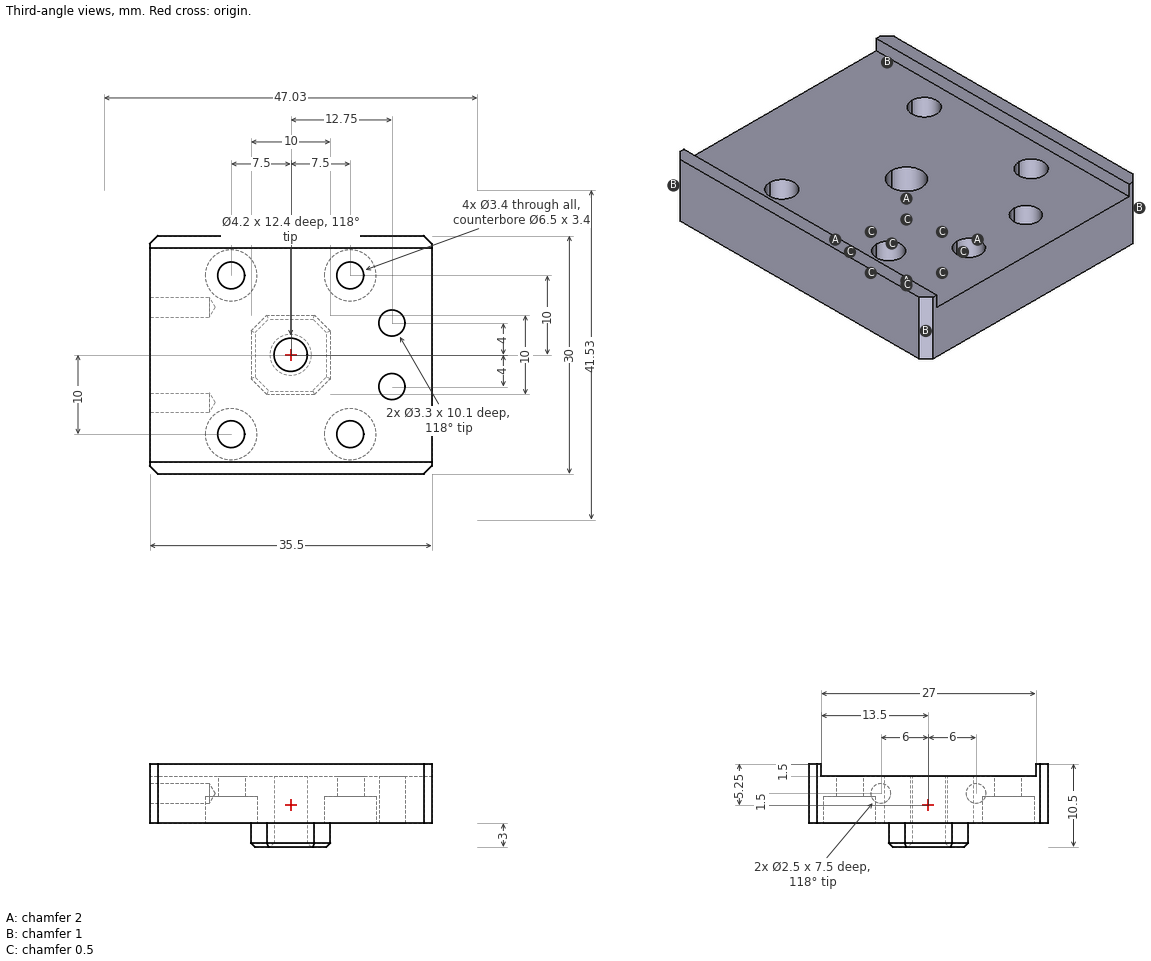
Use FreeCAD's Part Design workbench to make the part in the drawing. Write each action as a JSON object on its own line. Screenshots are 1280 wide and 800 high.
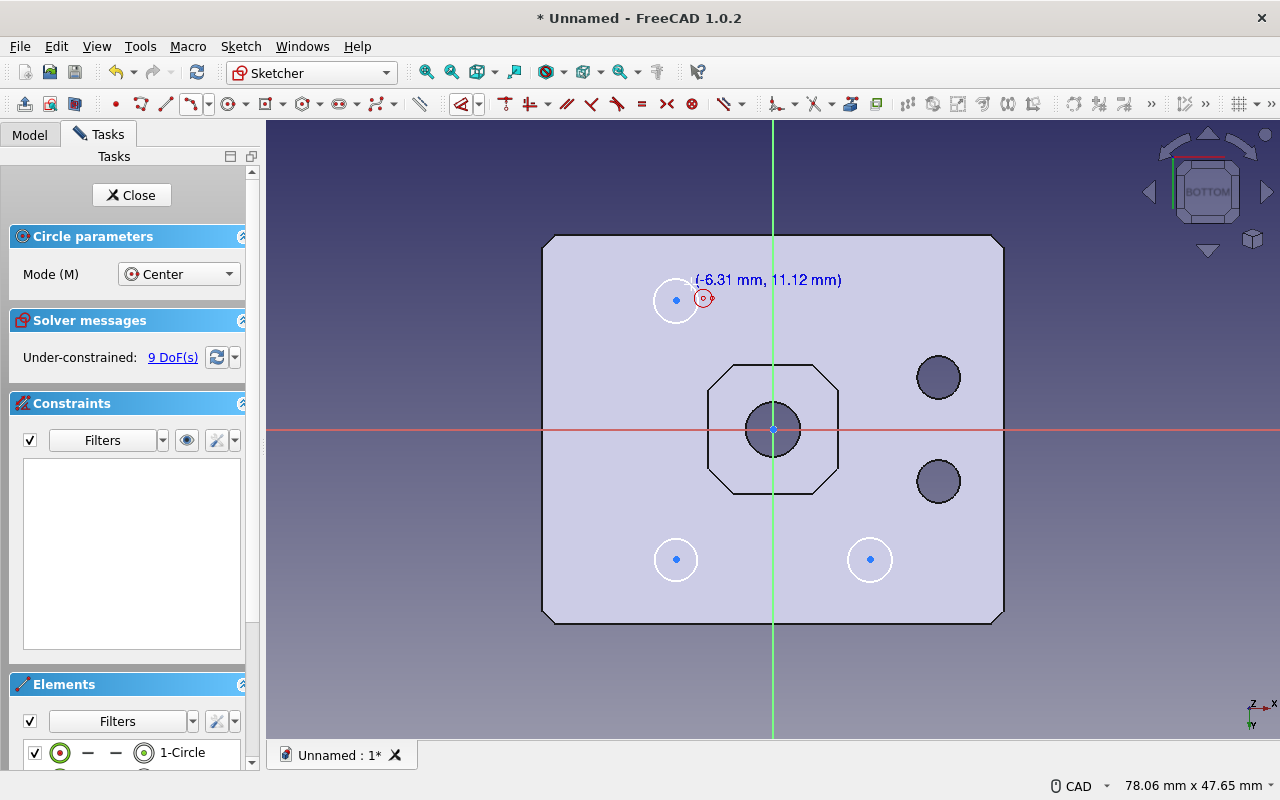
{"action": "left_click", "coordinate": [870, 300]}
{"action": "left_click", "coordinate": [886, 284]}
{"action": "key", "text": "Escape"}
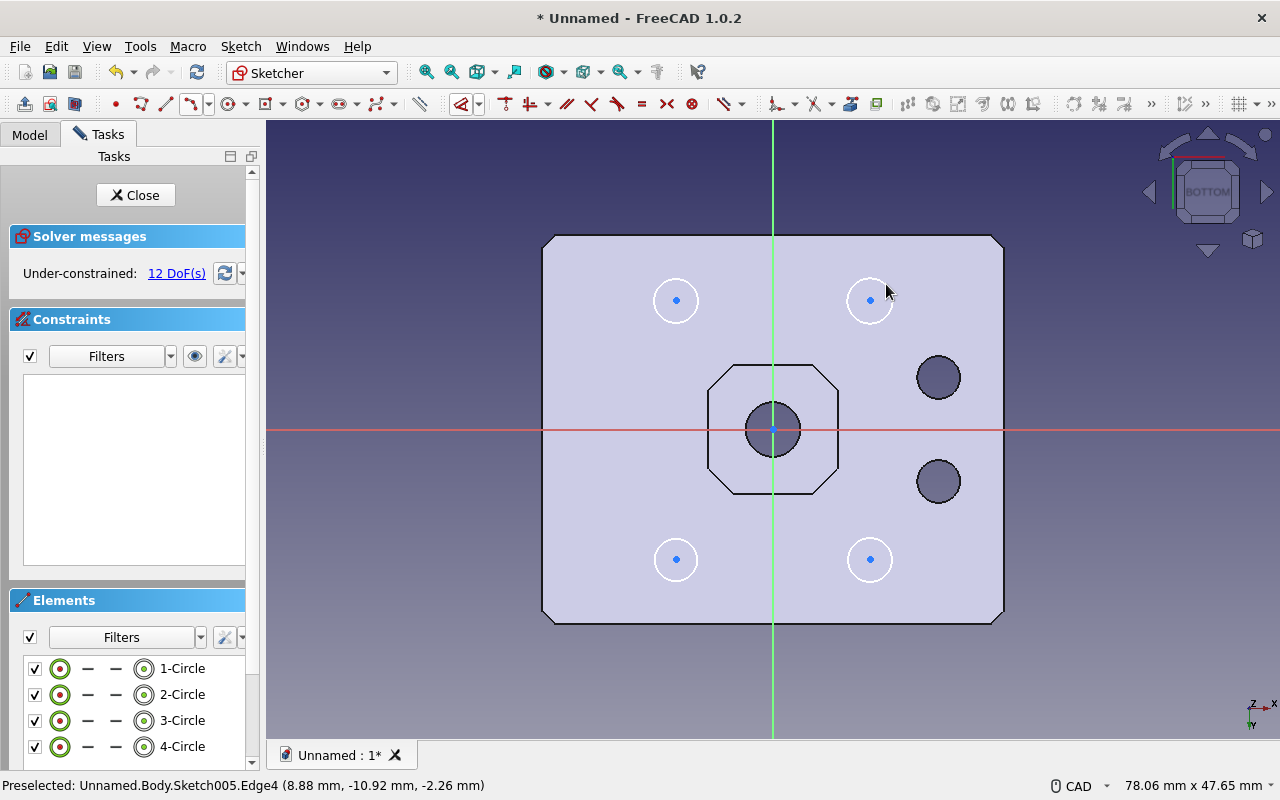
{"action": "left_click", "coordinate": [885, 544]}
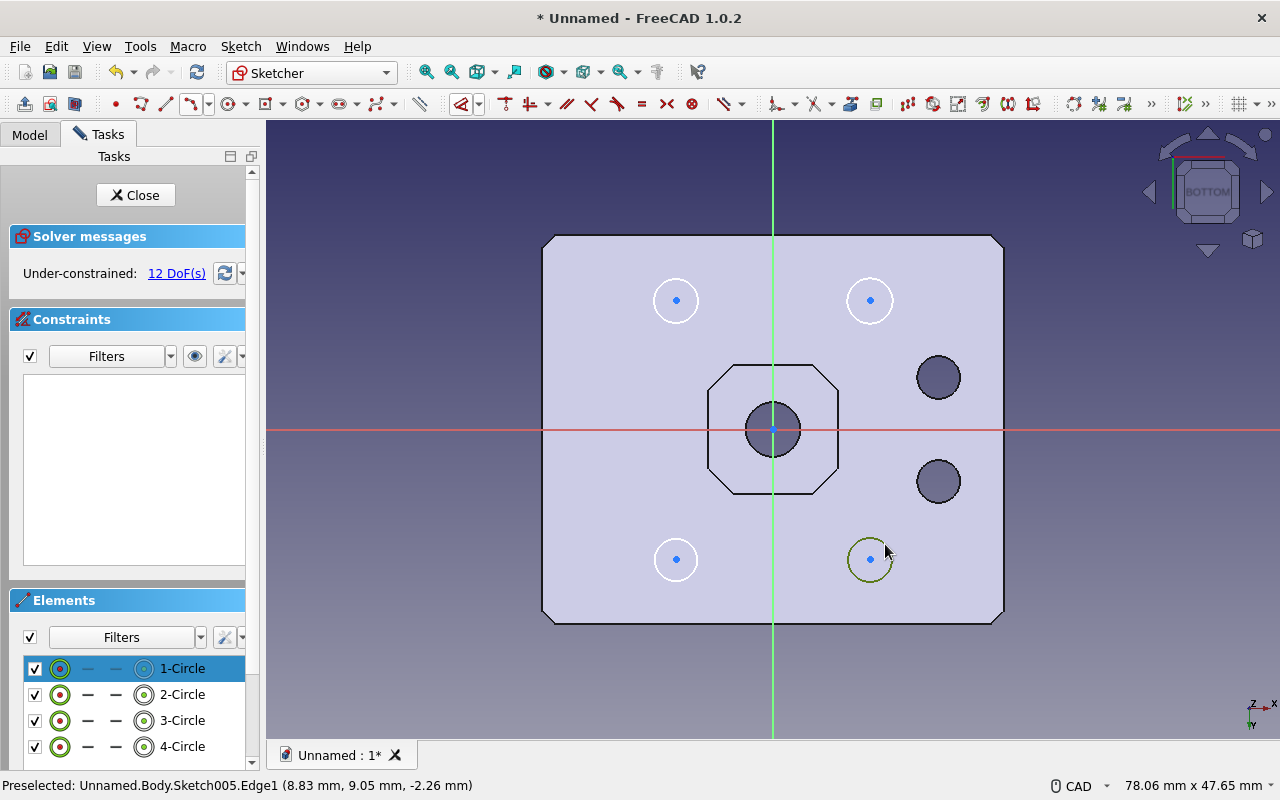
{"action": "left_click", "coordinate": [691, 545]}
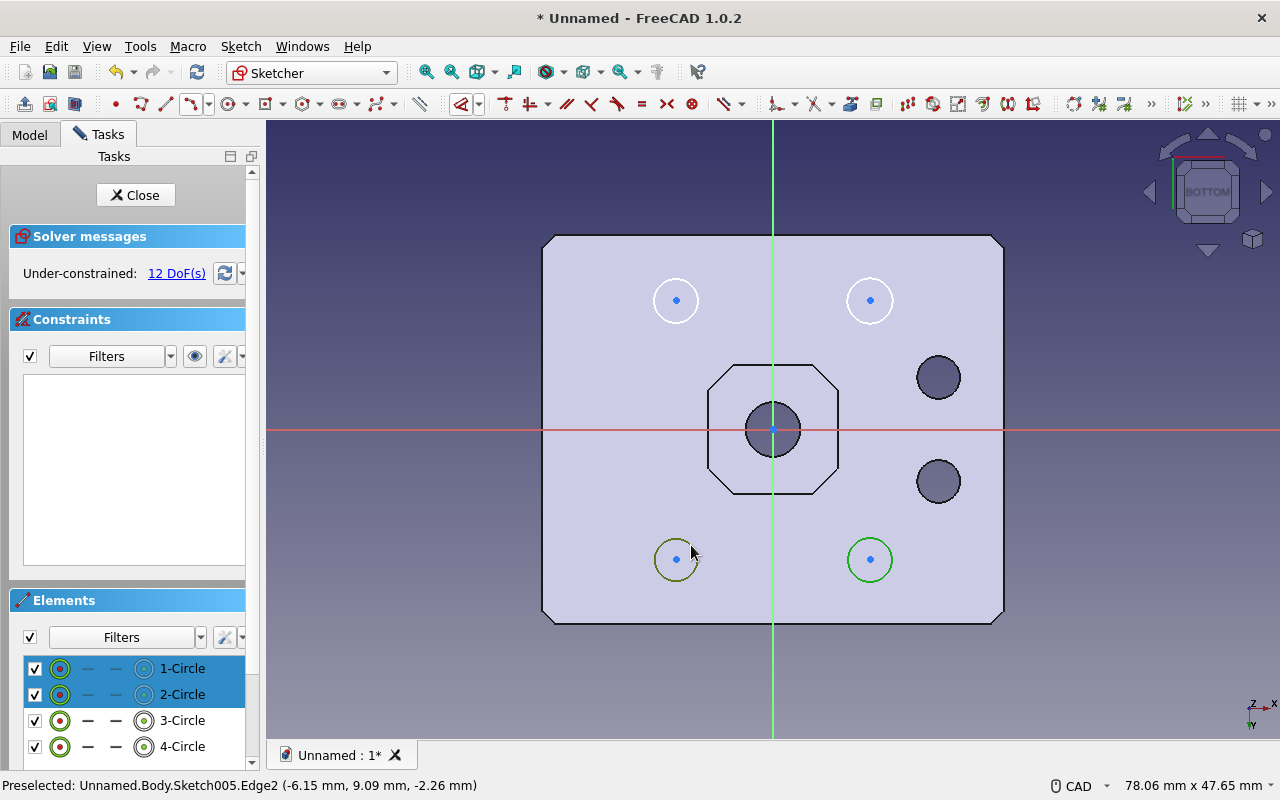
{"action": "left_click", "coordinate": [691, 285]}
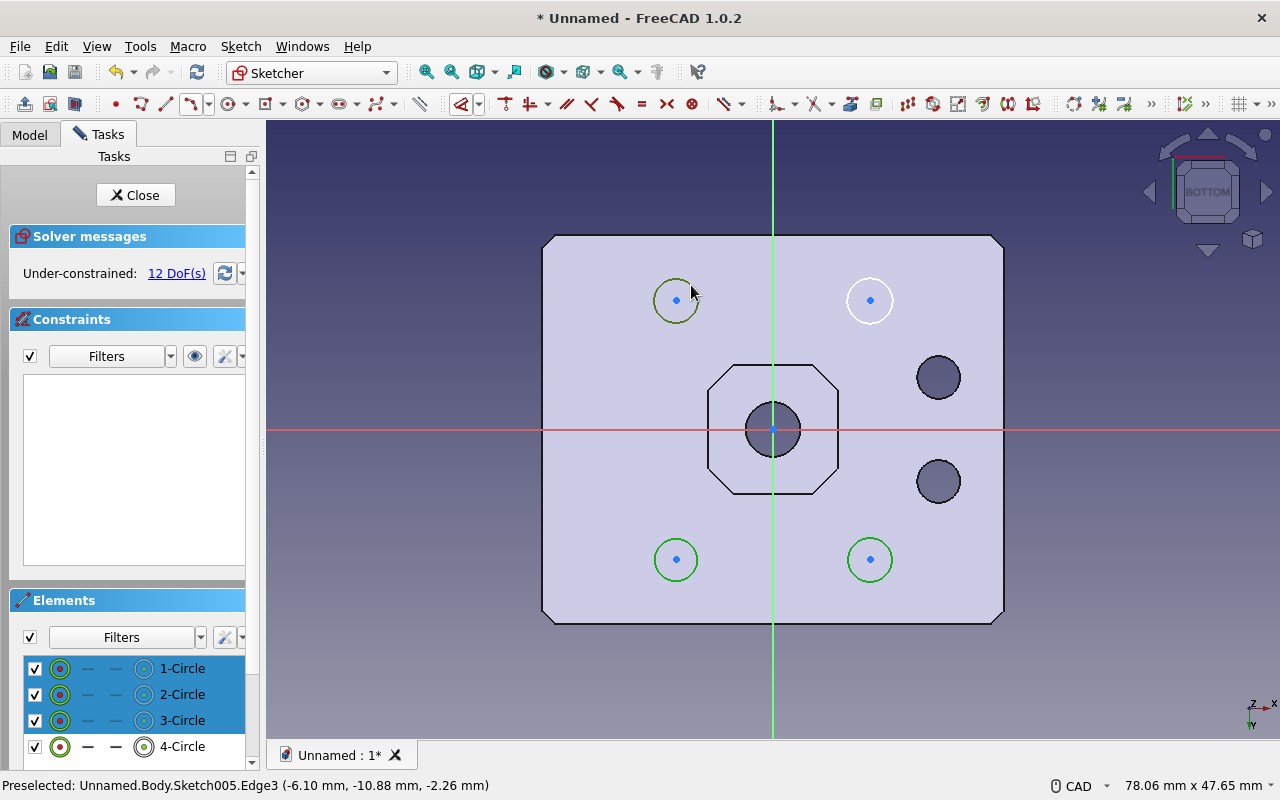
{"action": "left_click", "coordinate": [886, 285]}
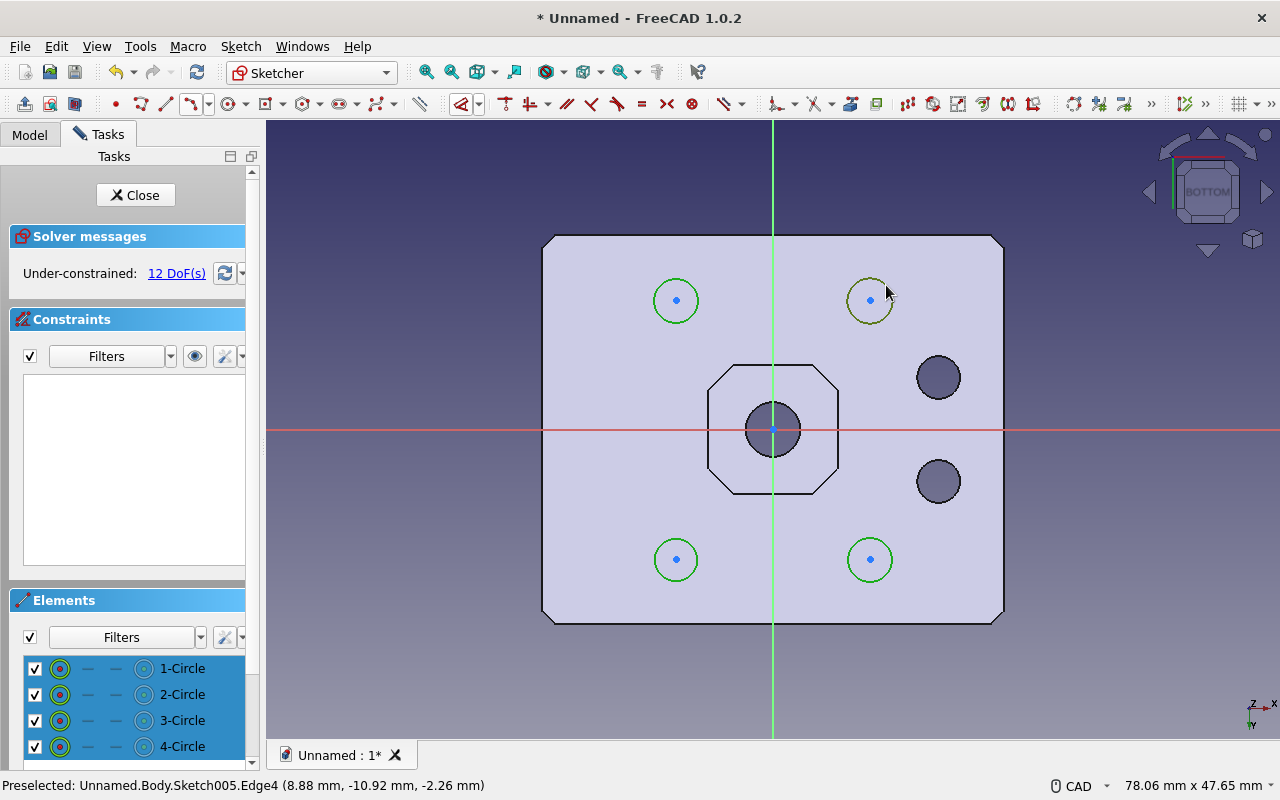
{"action": "left_click", "coordinate": [642, 104]}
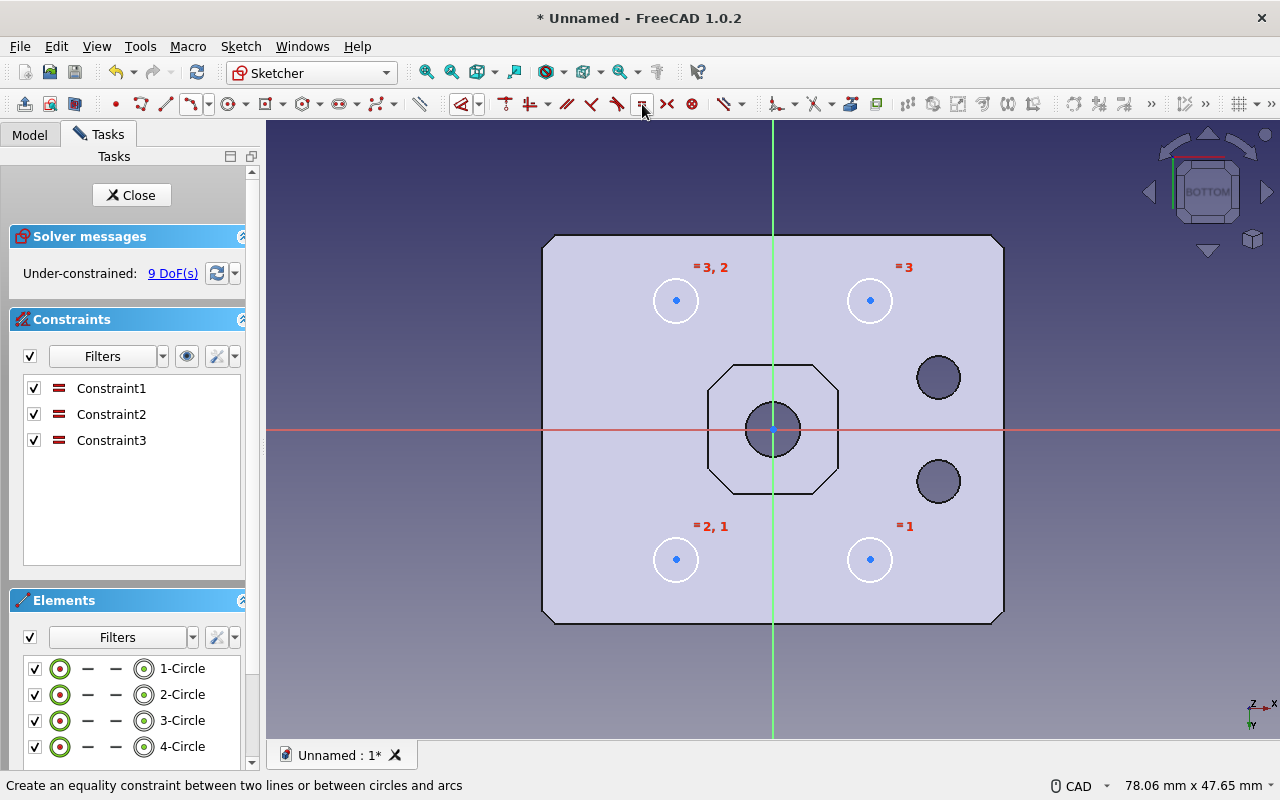
{"action": "left_click", "coordinate": [870, 560]}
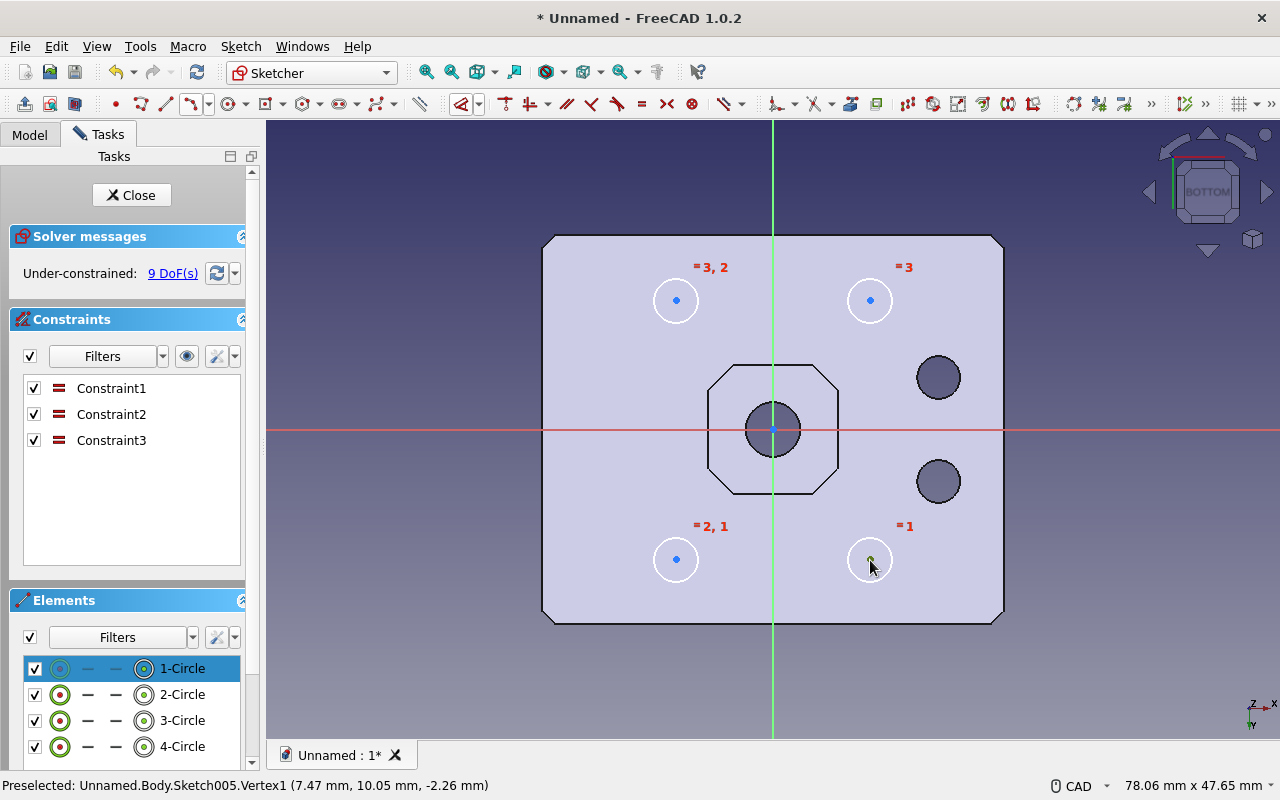
{"action": "left_click", "coordinate": [676, 560]}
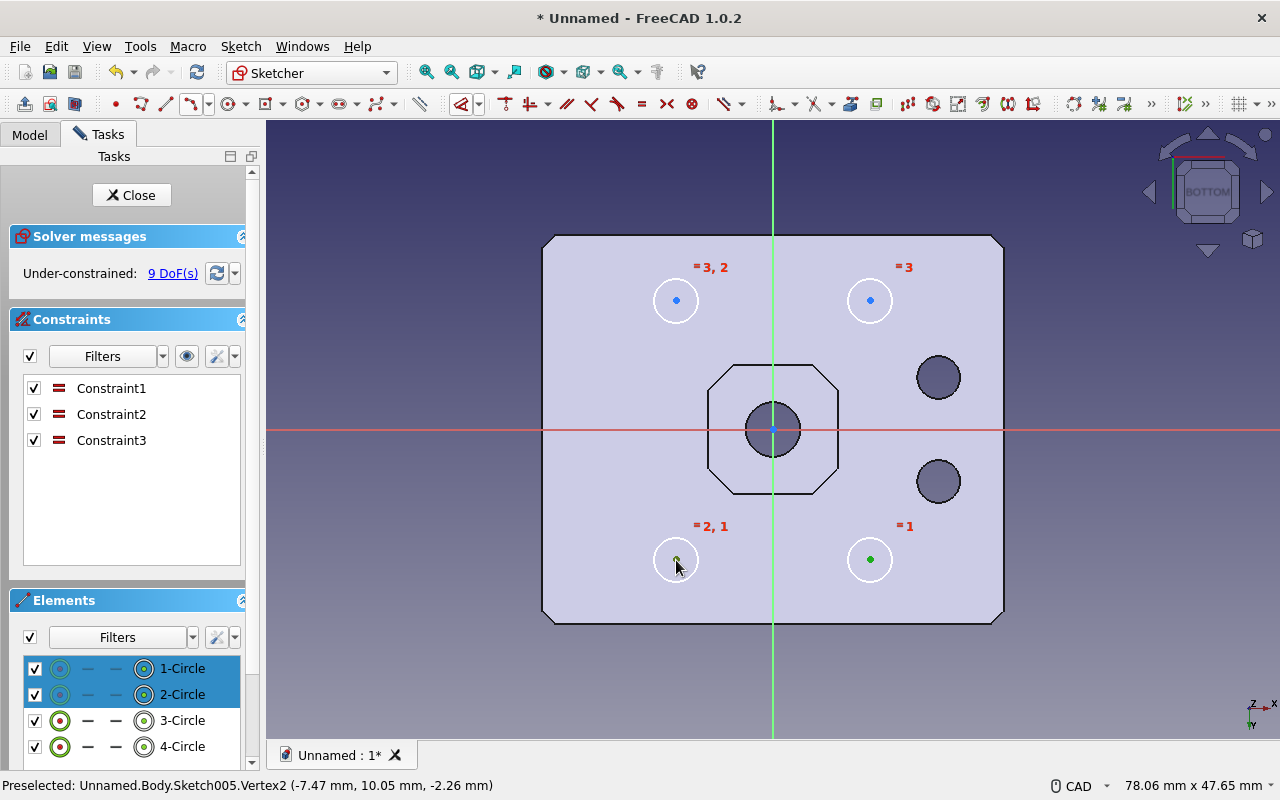
{"action": "key", "text": "h"}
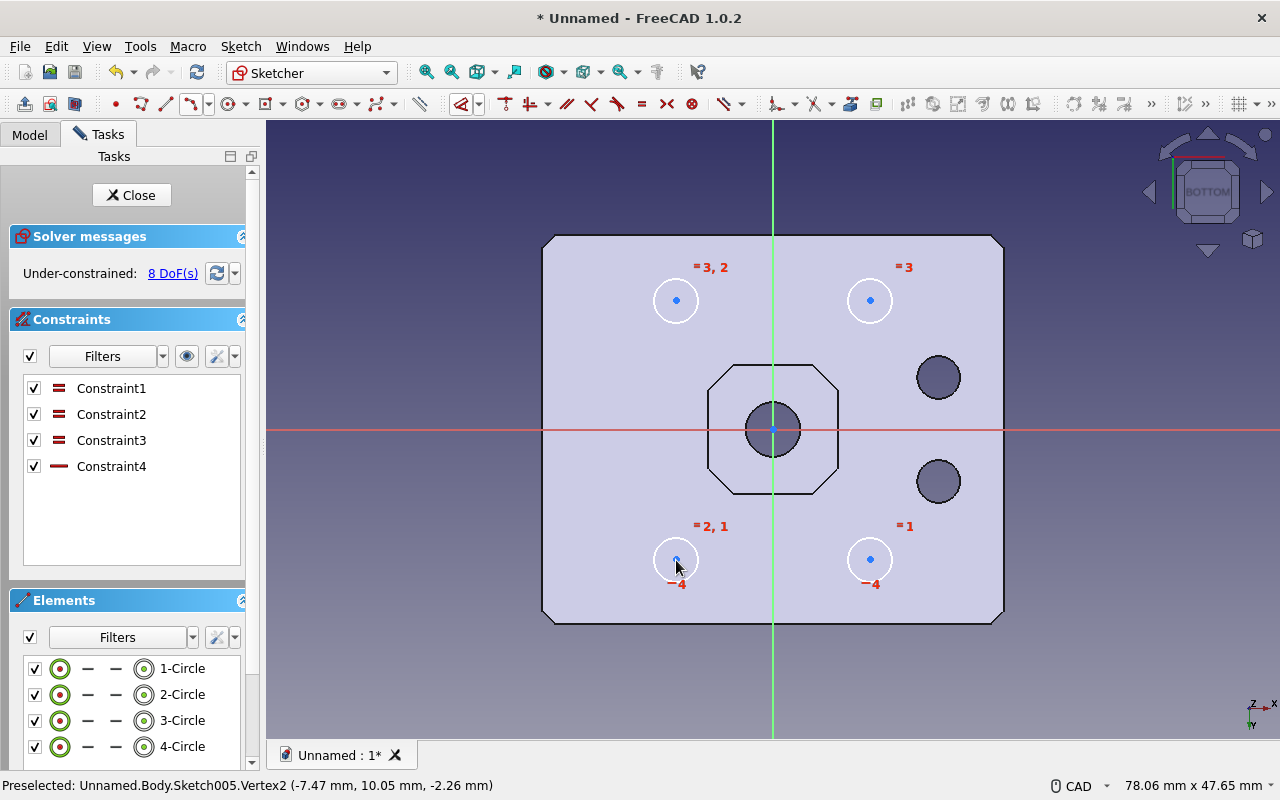
{"action": "left_click", "coordinate": [676, 560]}